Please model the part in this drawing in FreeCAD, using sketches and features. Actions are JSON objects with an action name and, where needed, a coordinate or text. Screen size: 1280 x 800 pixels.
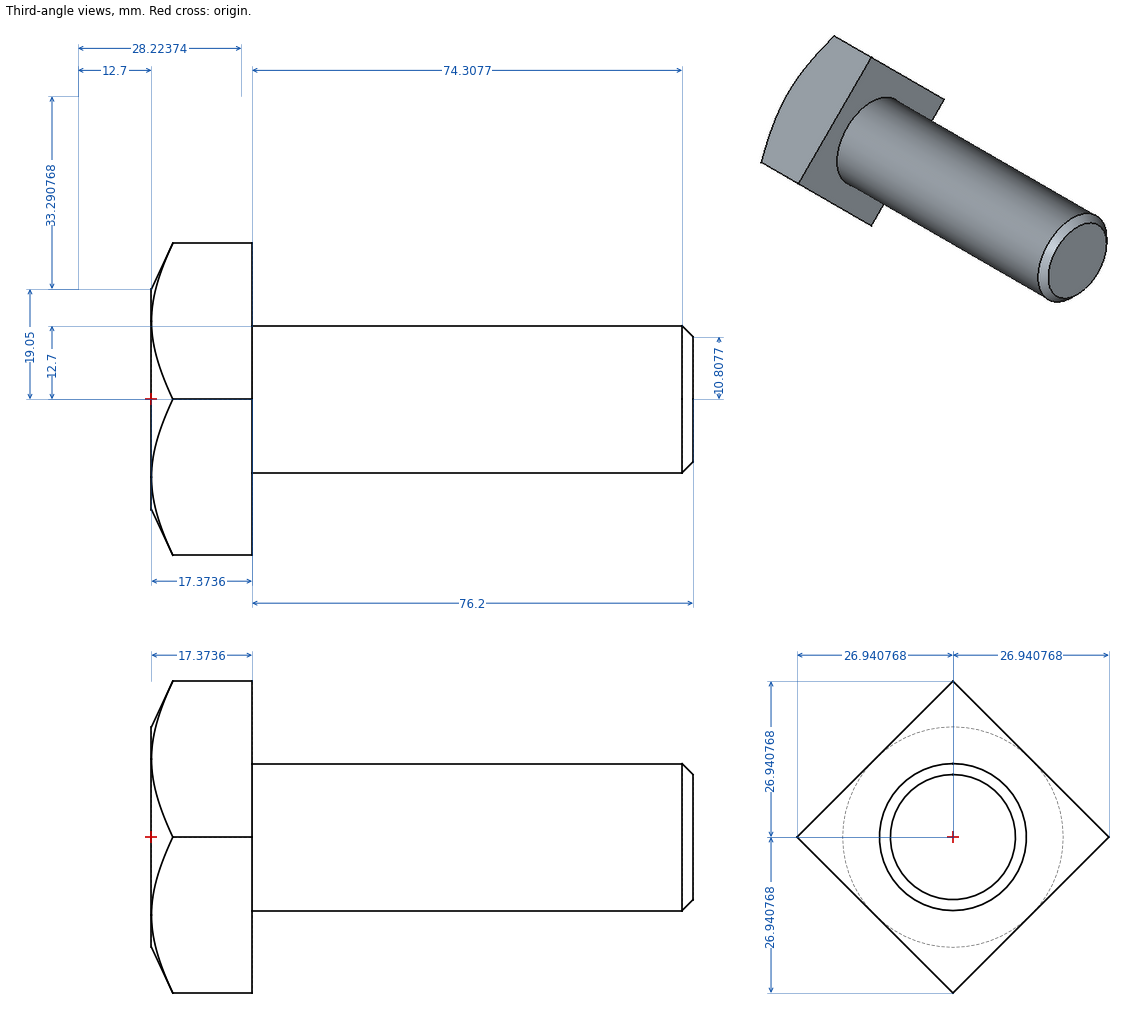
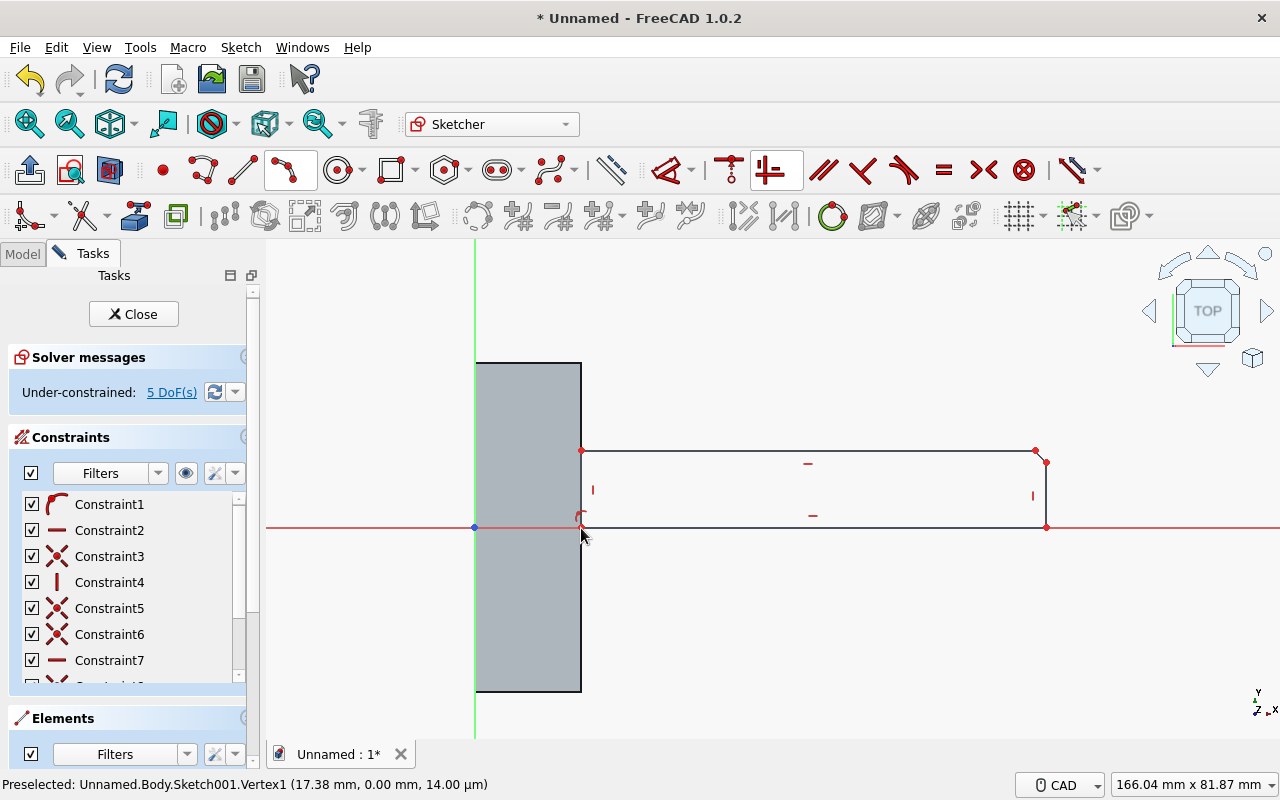
{"action": "key", "text": "d"}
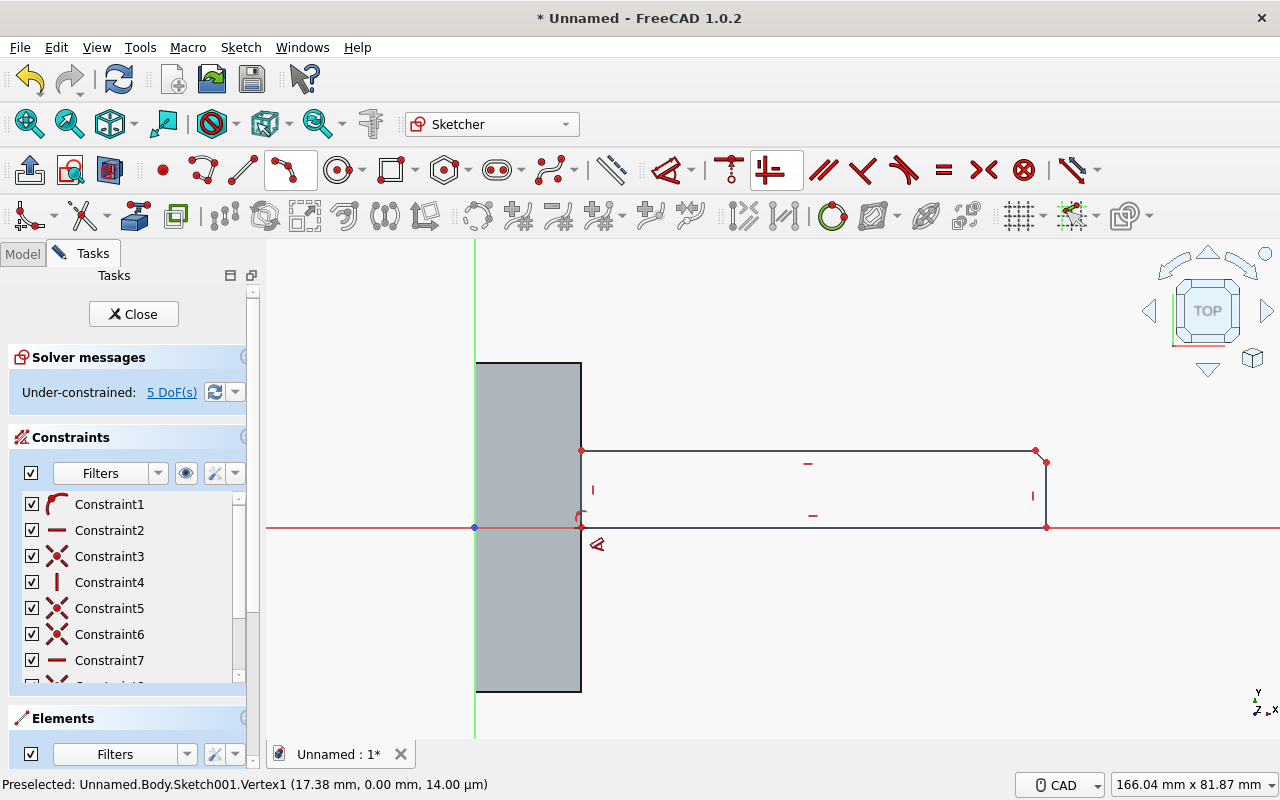
{"action": "left_click", "coordinate": [720, 528]}
{"action": "left_click", "coordinate": [813, 562]}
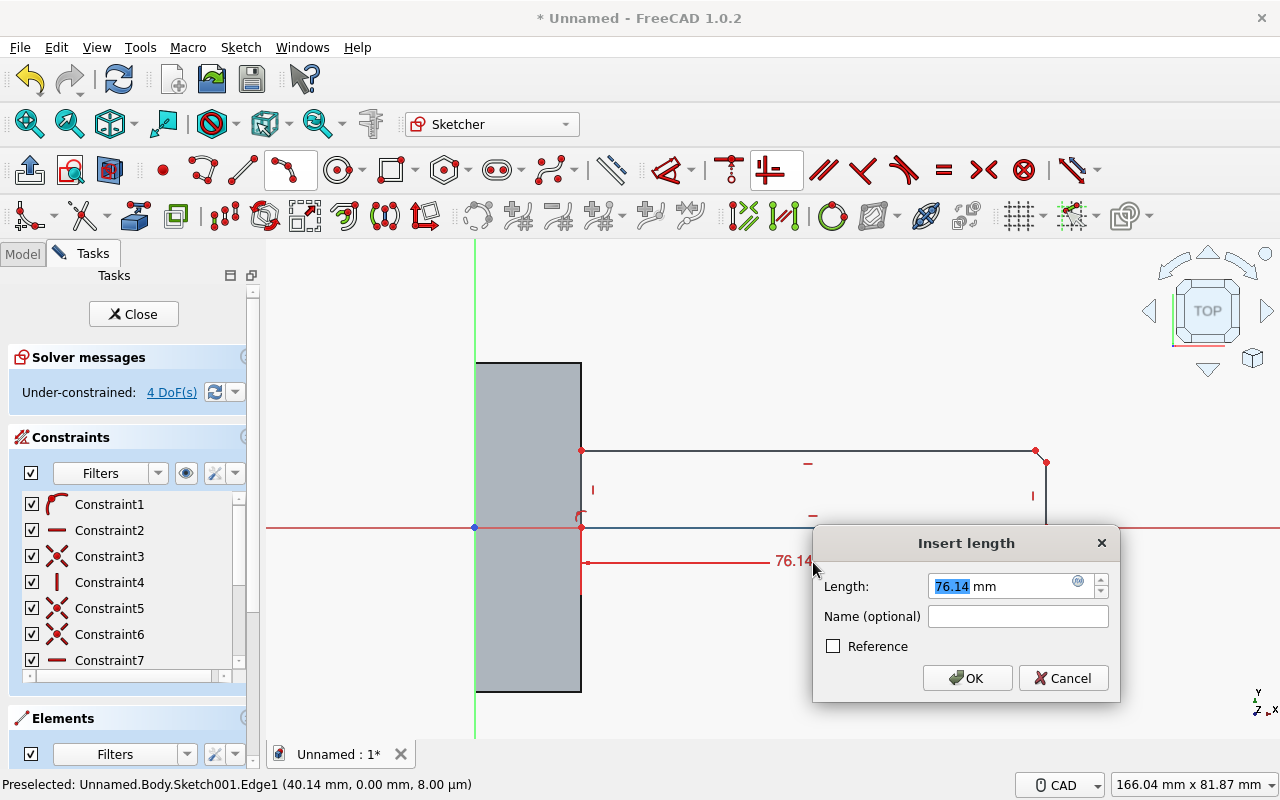
{"action": "type", "text": "76.2"}
{"action": "key", "text": "Return"}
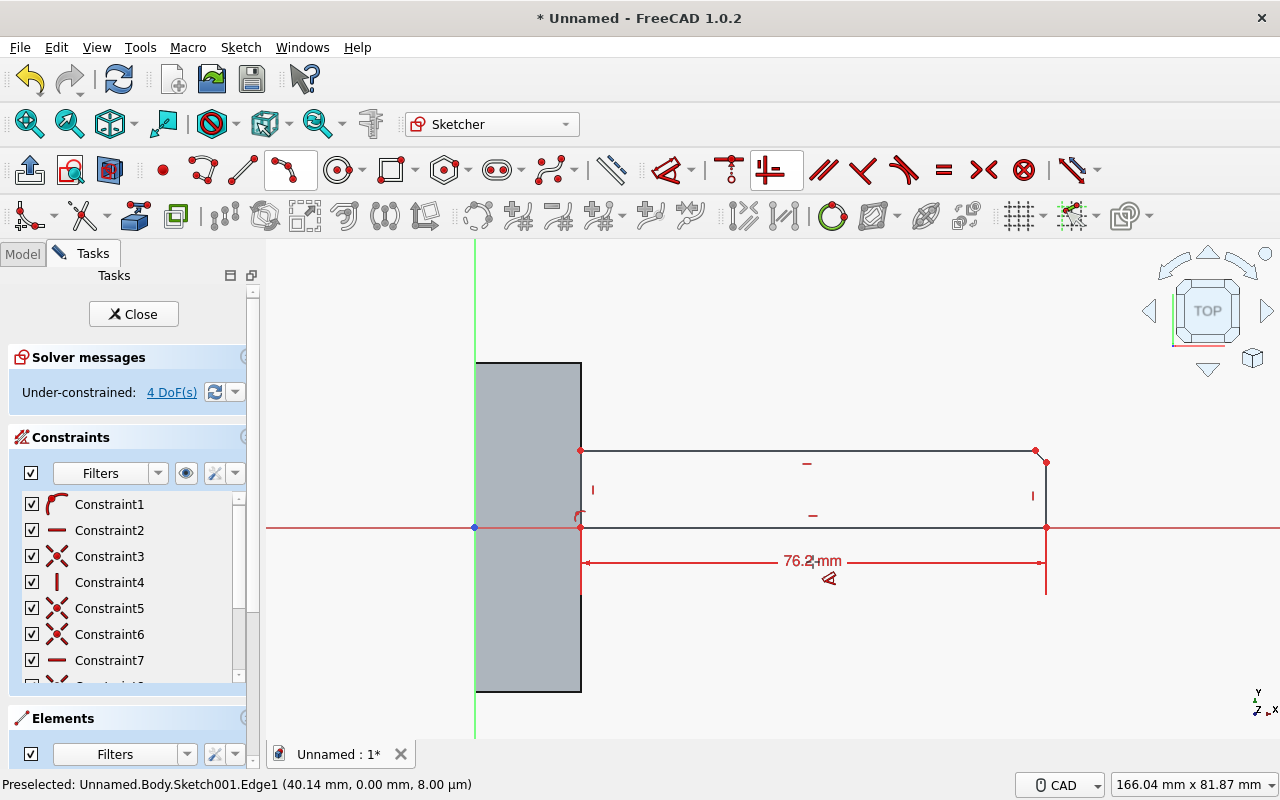
{"action": "left_click", "coordinate": [581, 474]}
{"action": "left_click", "coordinate": [547, 489]}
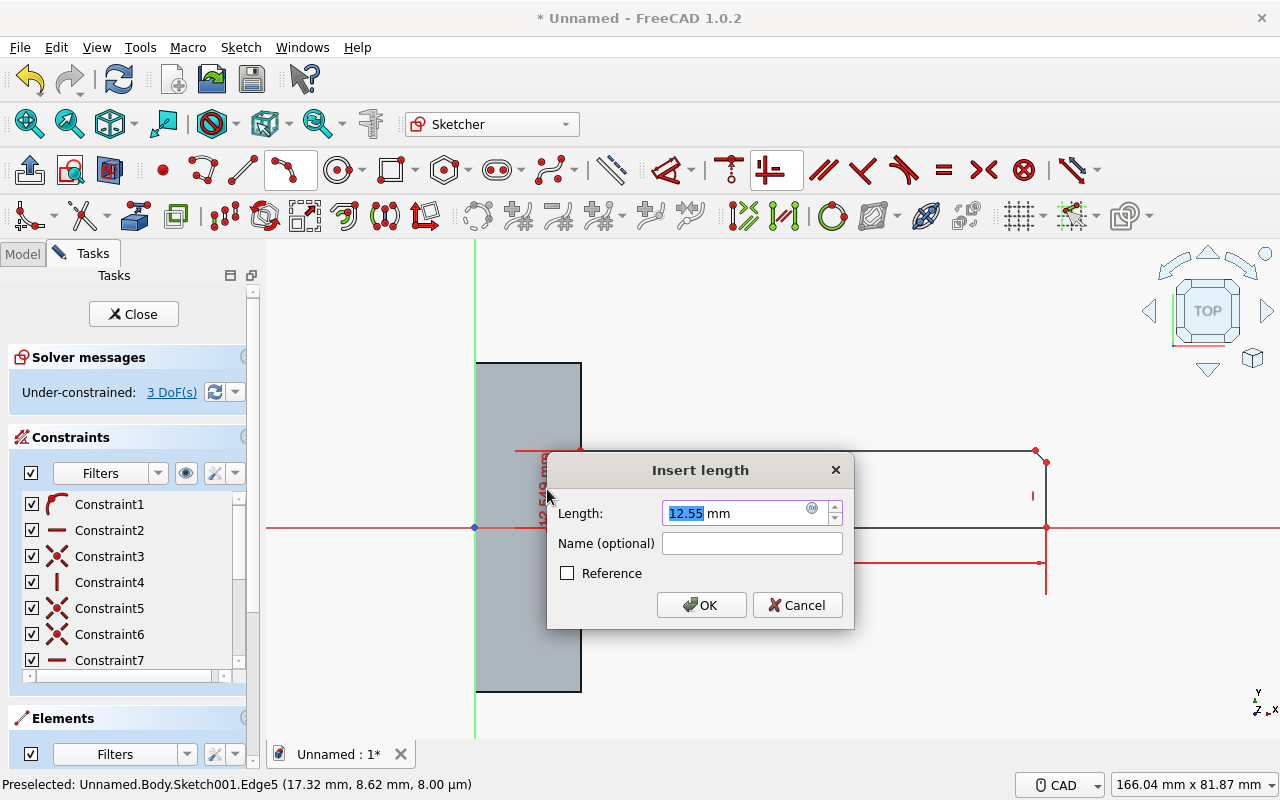
{"action": "type", "text": "12.7"}
{"action": "key", "text": "Return"}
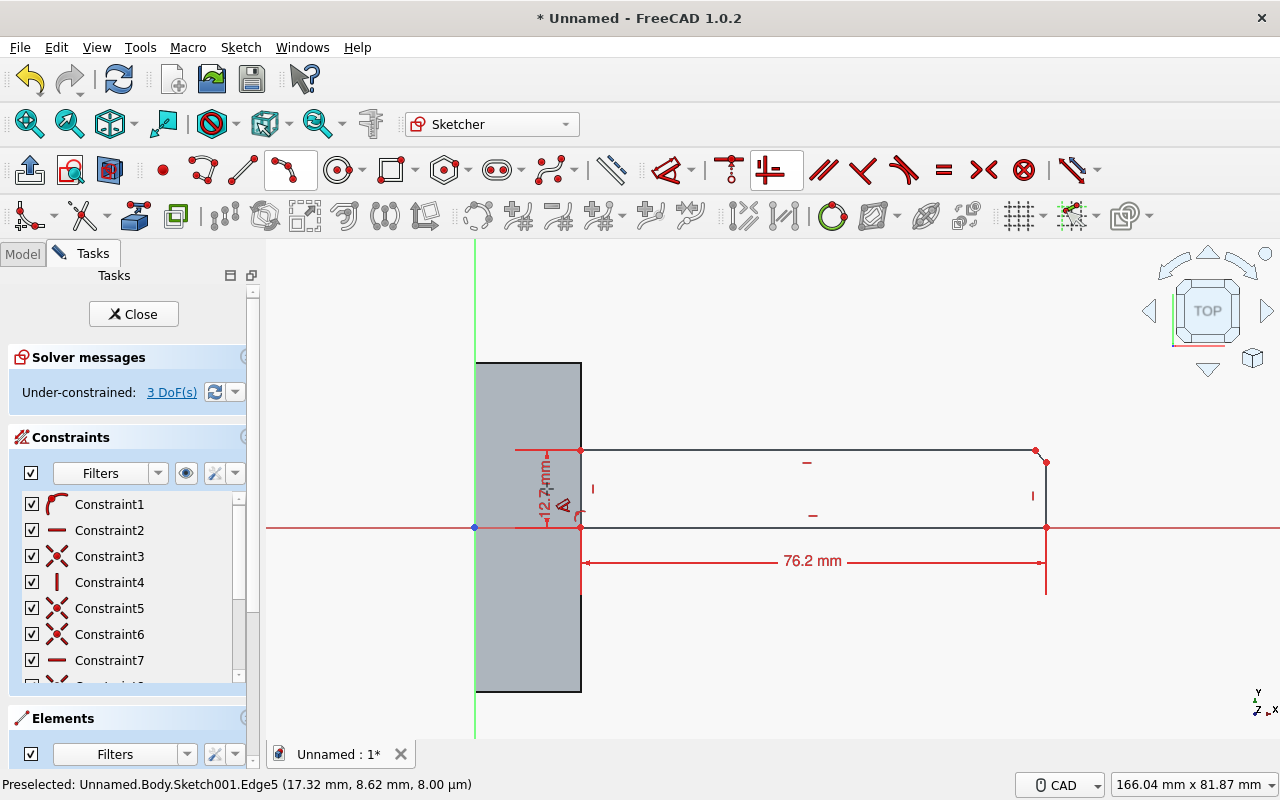
{"action": "left_click", "coordinate": [1046, 508]}
{"action": "left_click", "coordinate": [1080, 495]}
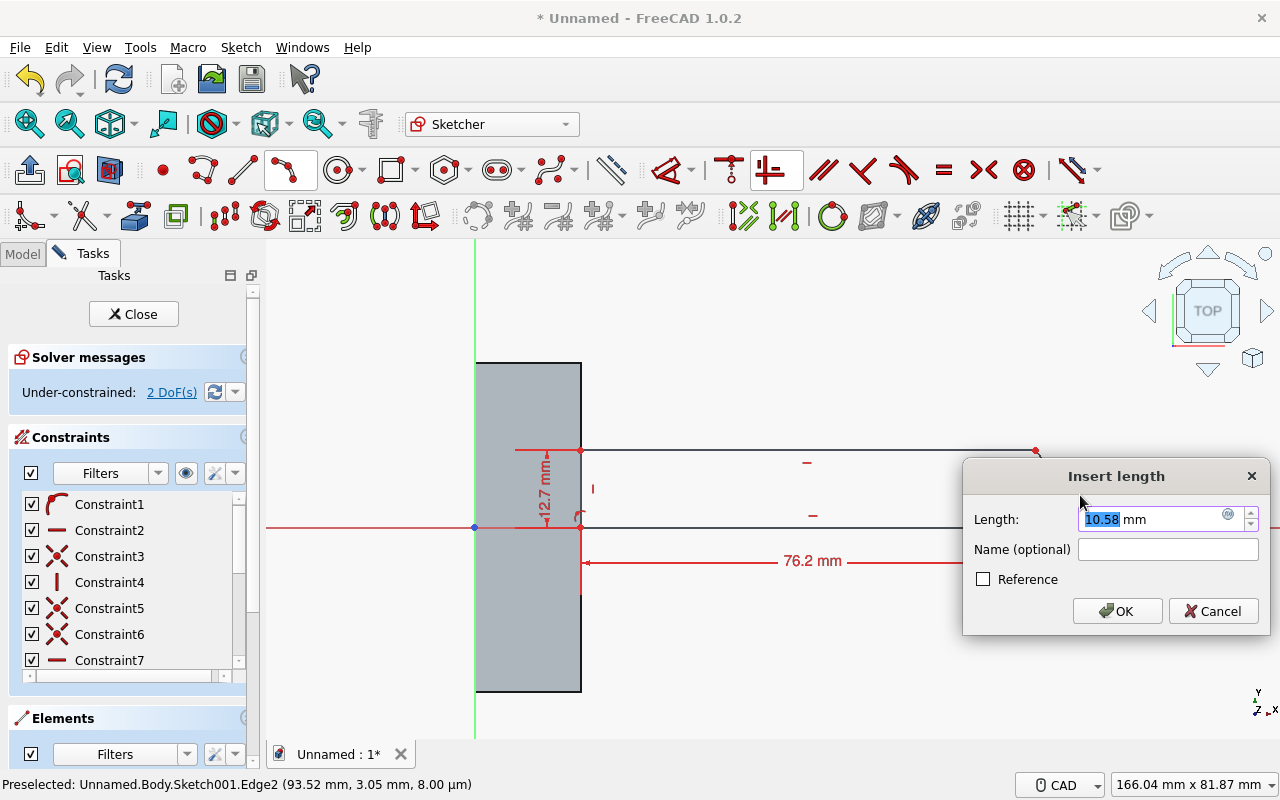
{"action": "type", "text": "10.8077"}
{"action": "key", "text": "Return"}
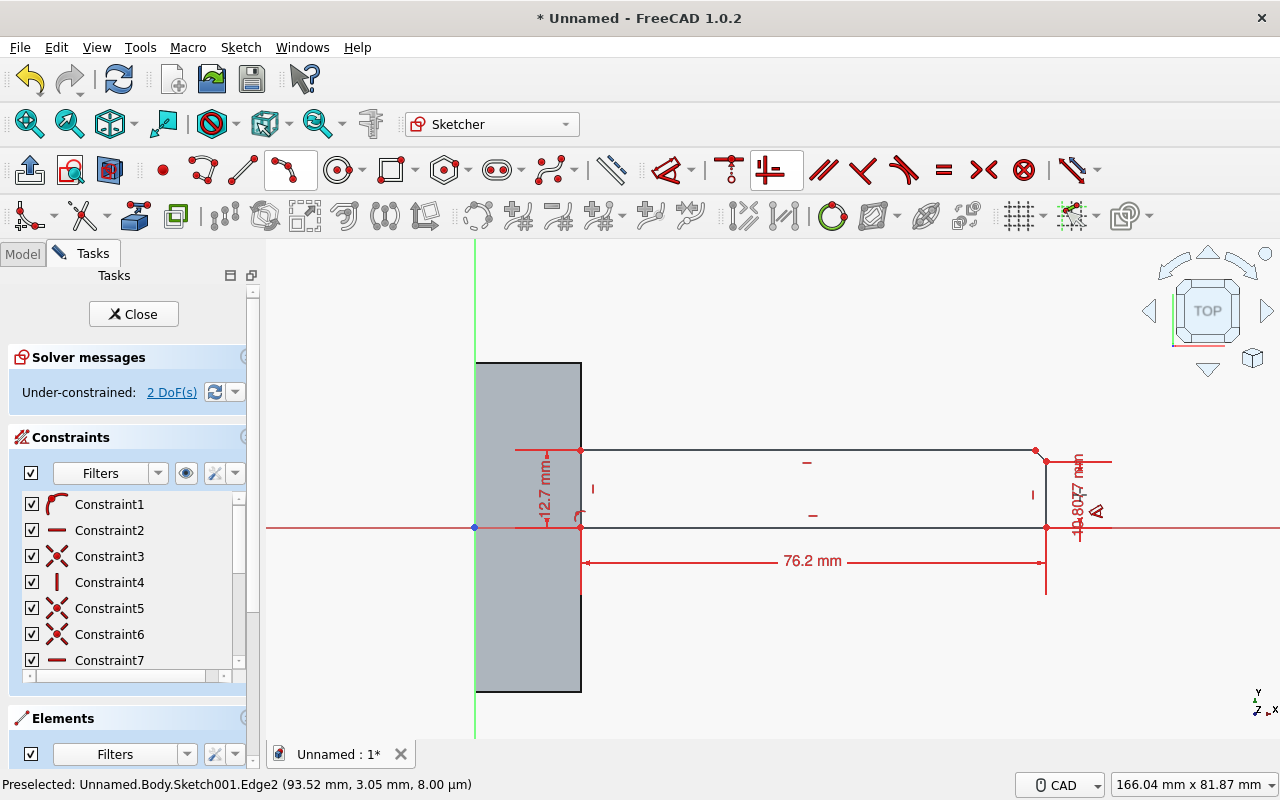
{"action": "left_click", "coordinate": [899, 450]}
{"action": "left_click", "coordinate": [808, 416]}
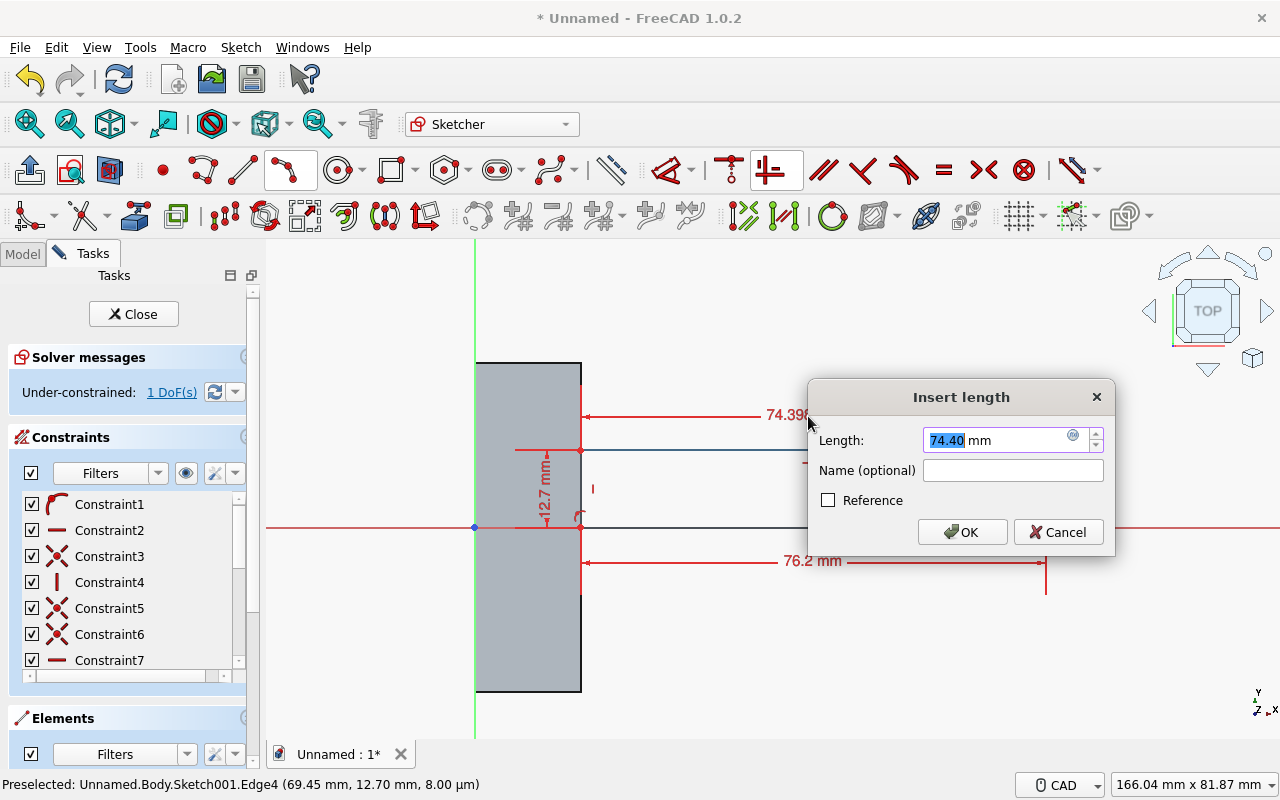
{"action": "type", "text": "74.3077"}
{"action": "key", "text": "Return"}